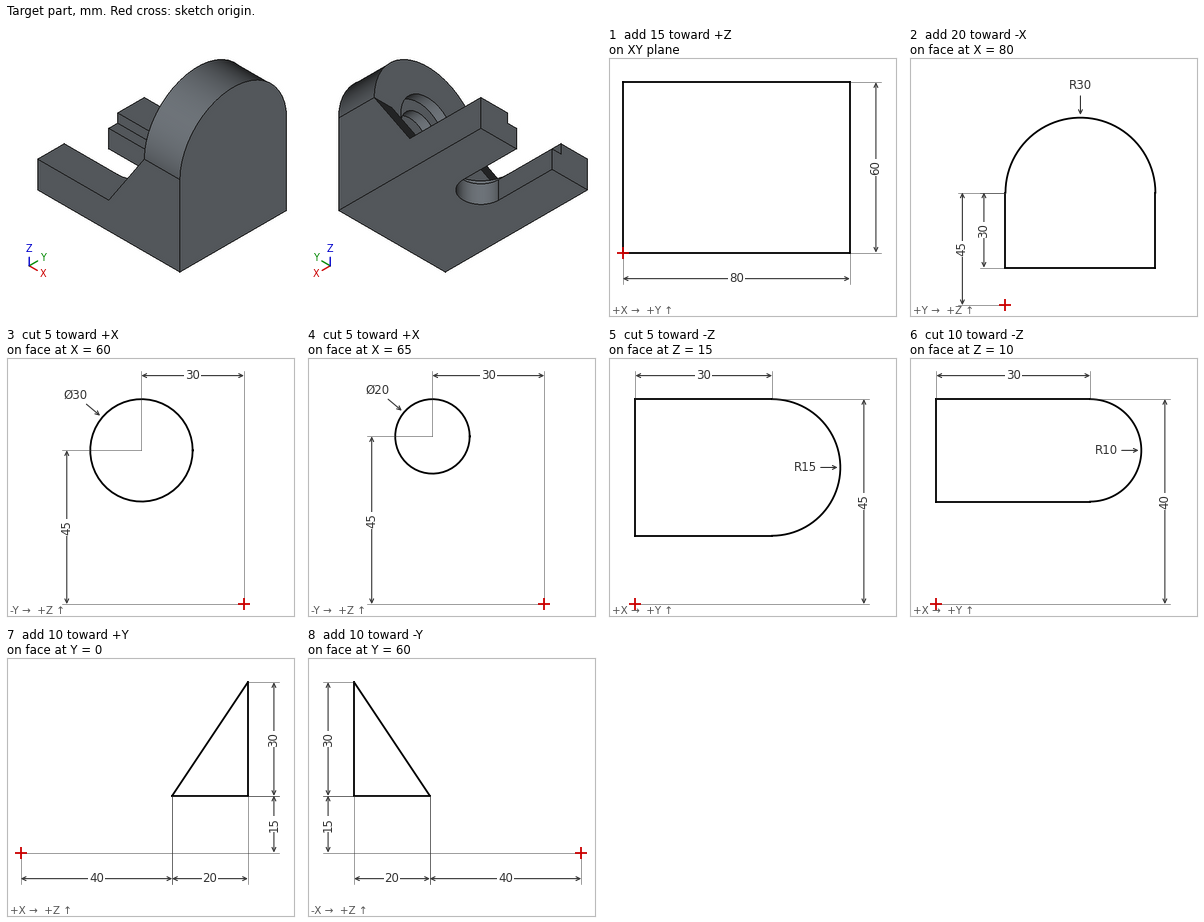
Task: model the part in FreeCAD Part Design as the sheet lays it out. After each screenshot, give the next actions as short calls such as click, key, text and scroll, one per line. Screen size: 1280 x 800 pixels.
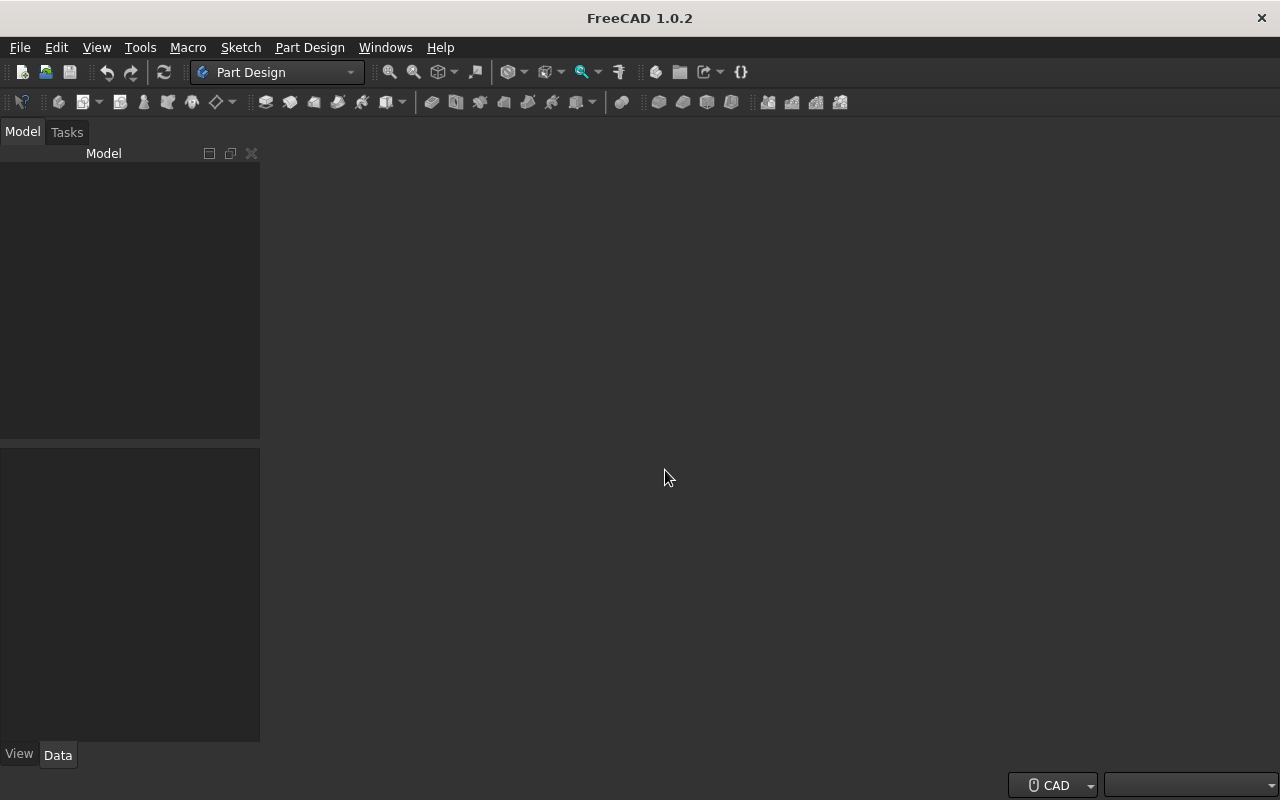
click(22, 72)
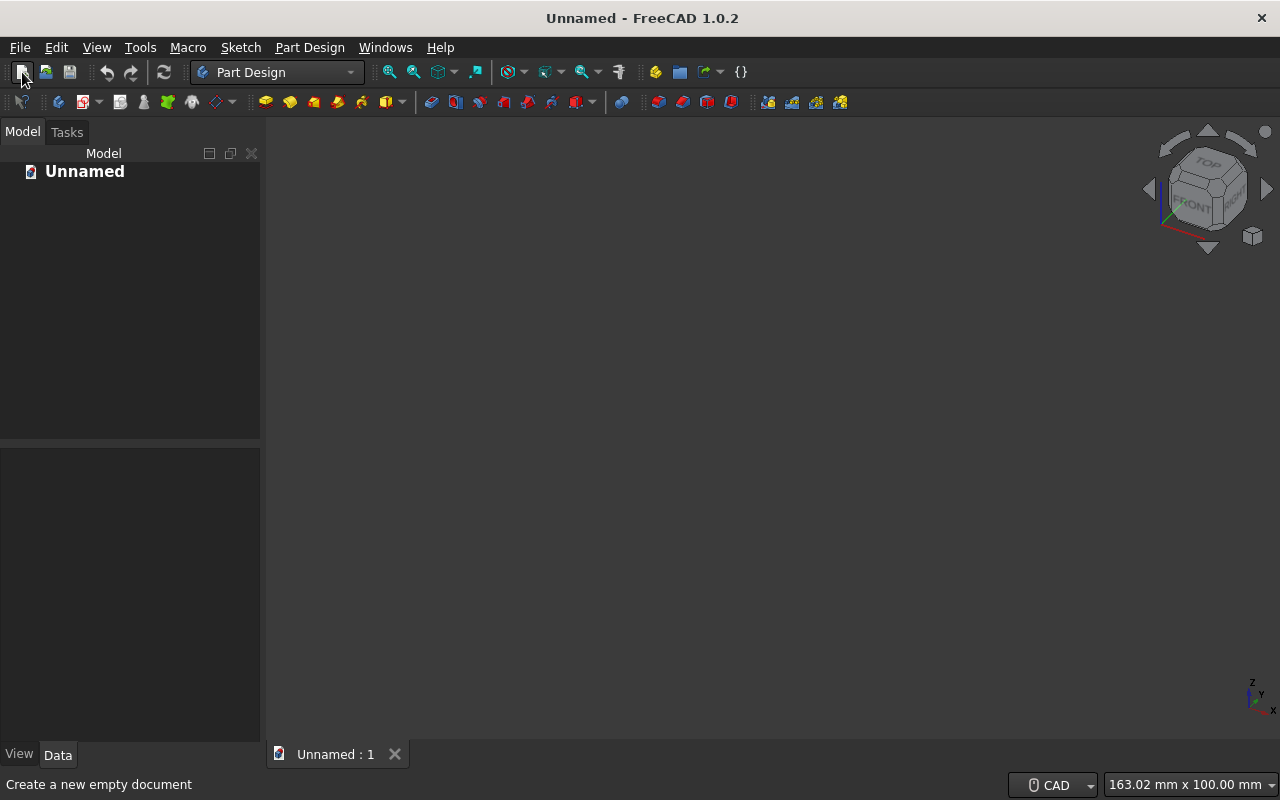
click(84, 102)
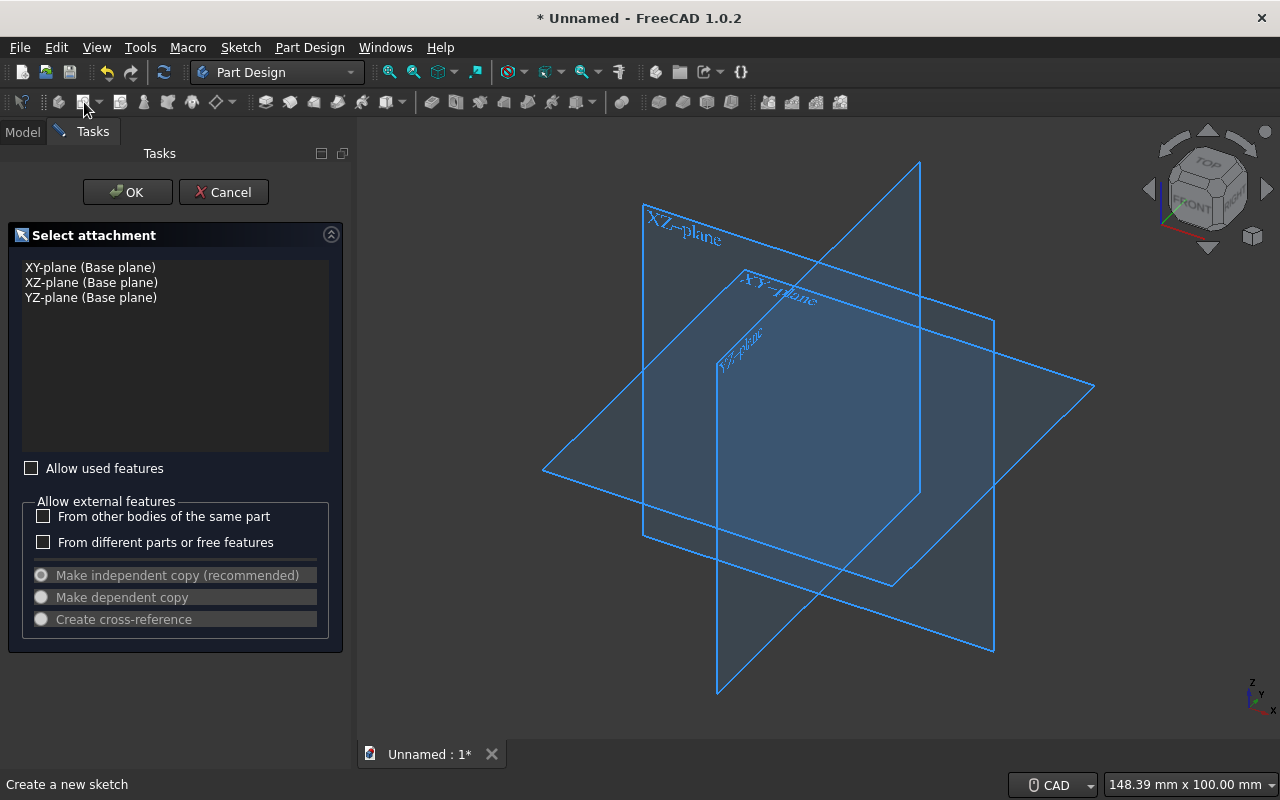
click(82, 268)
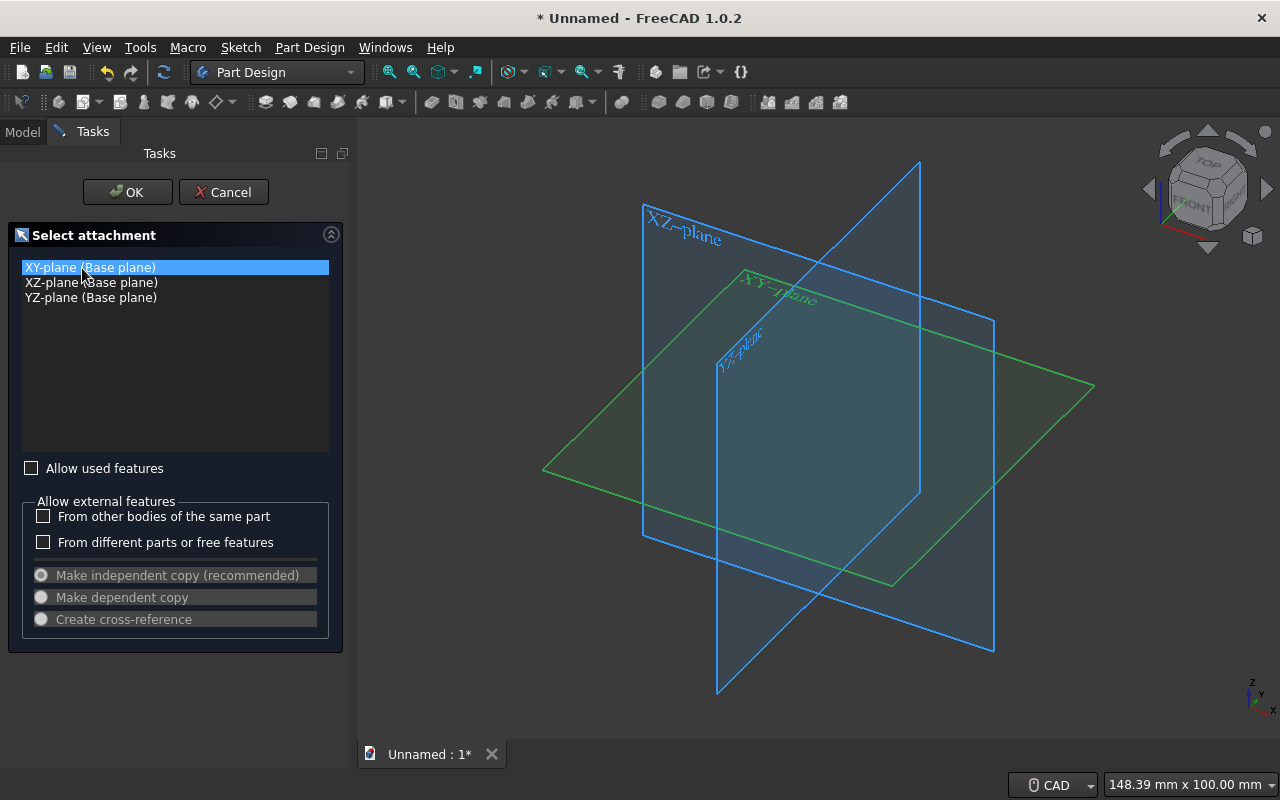
click(128, 192)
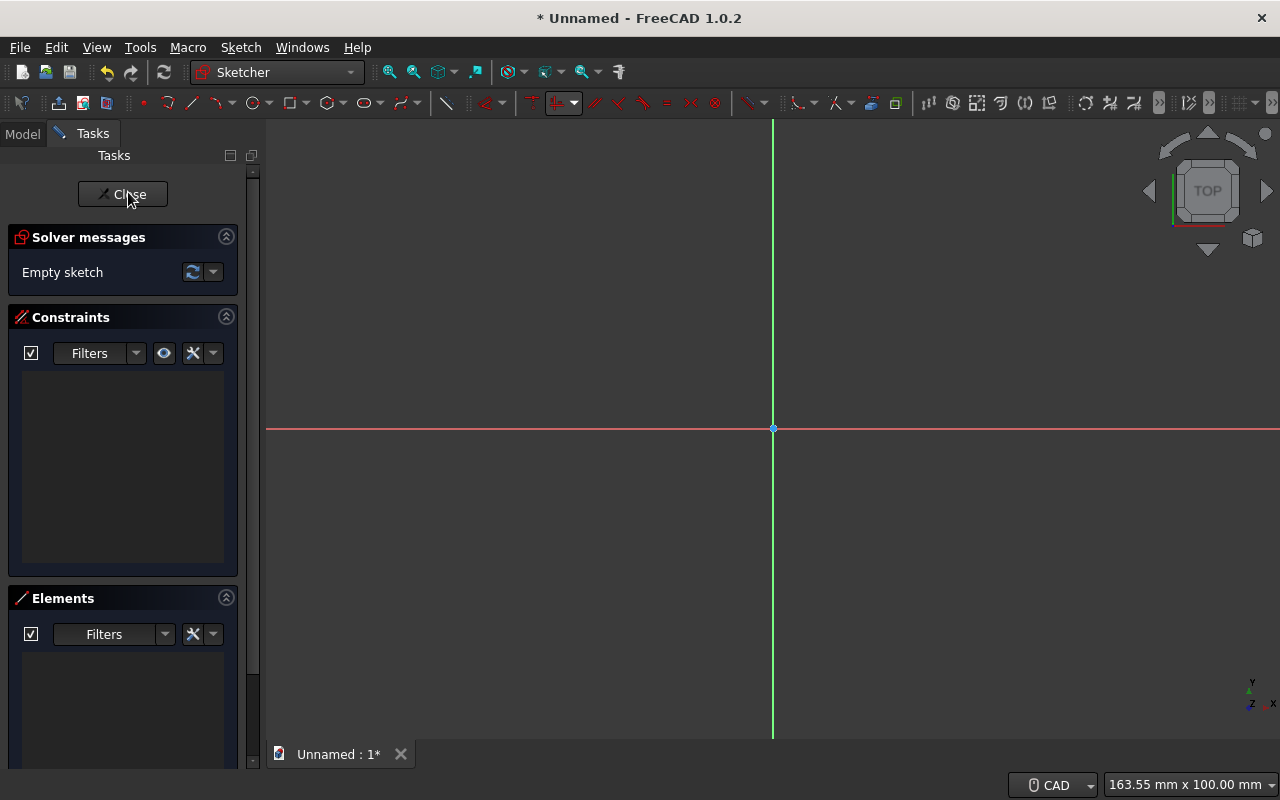
scroll(294, 711, down, 2)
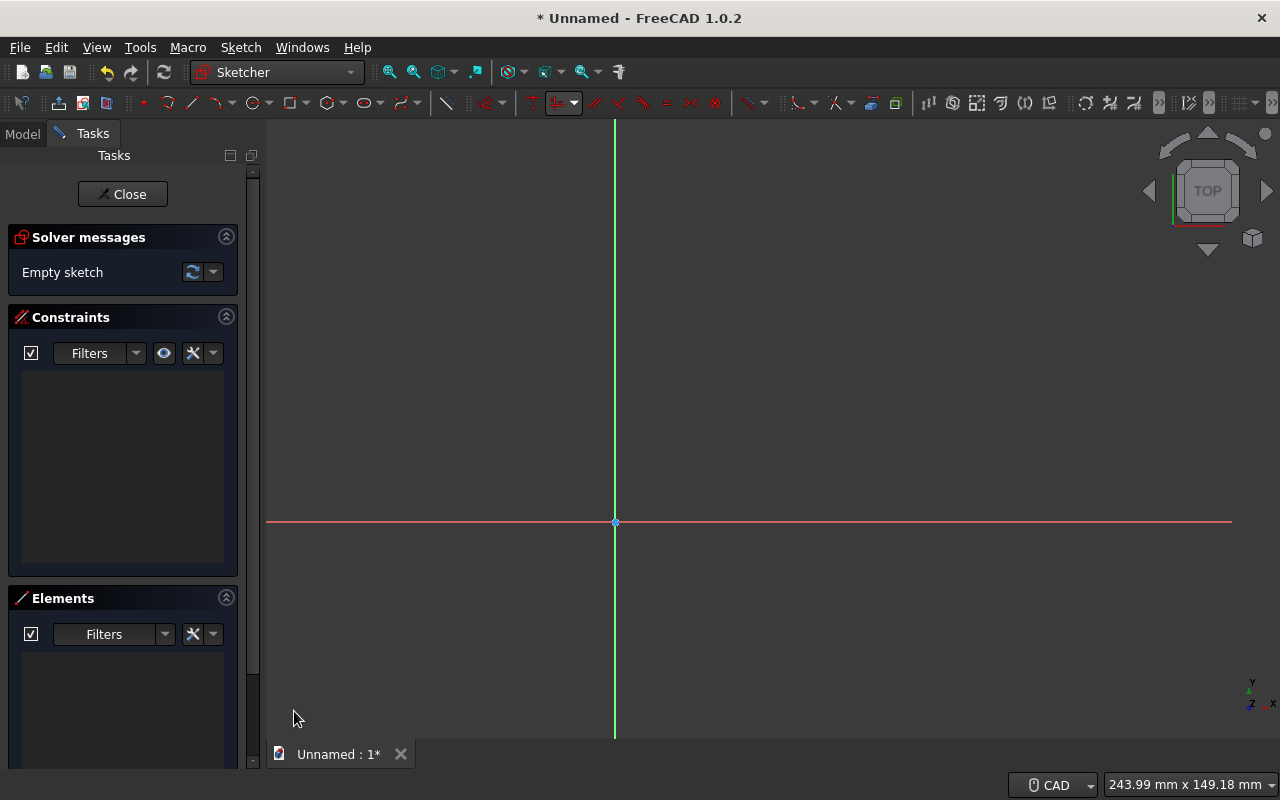
scroll(938, 334, up, 2)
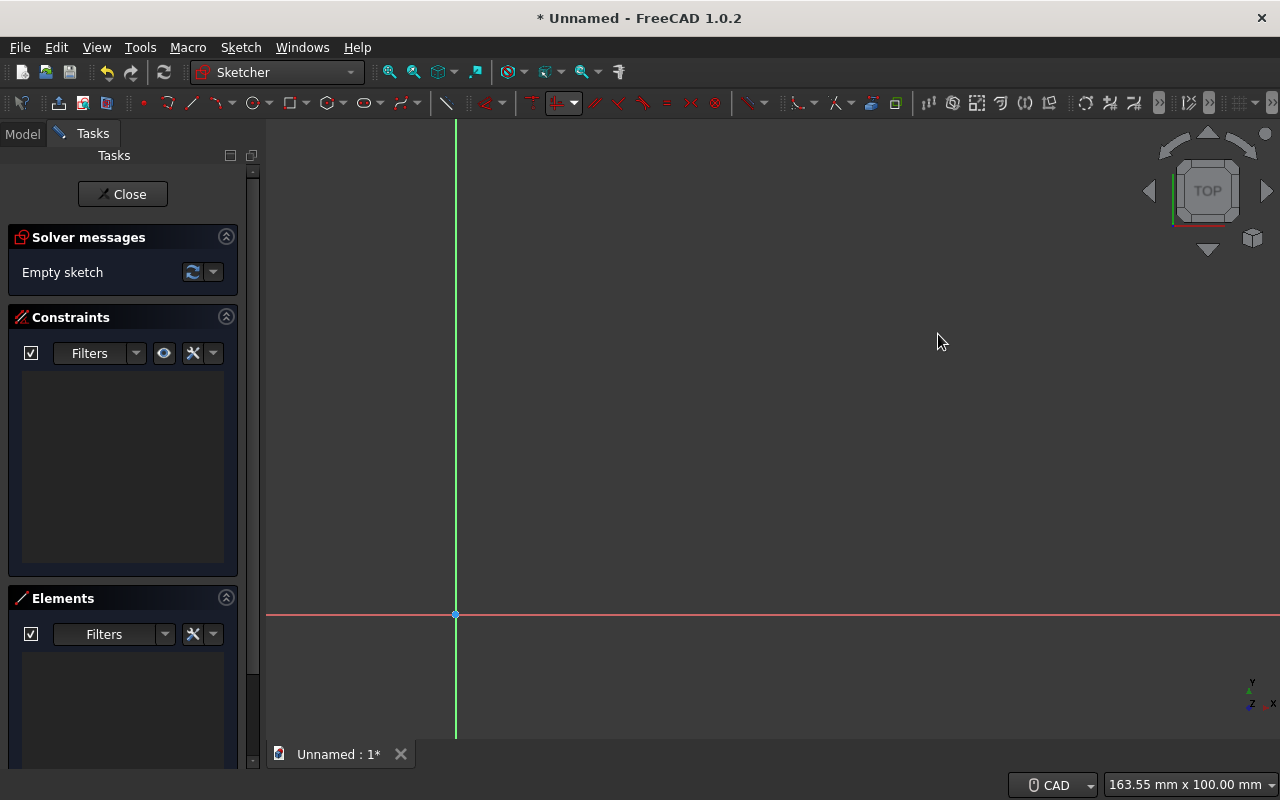
click(290, 104)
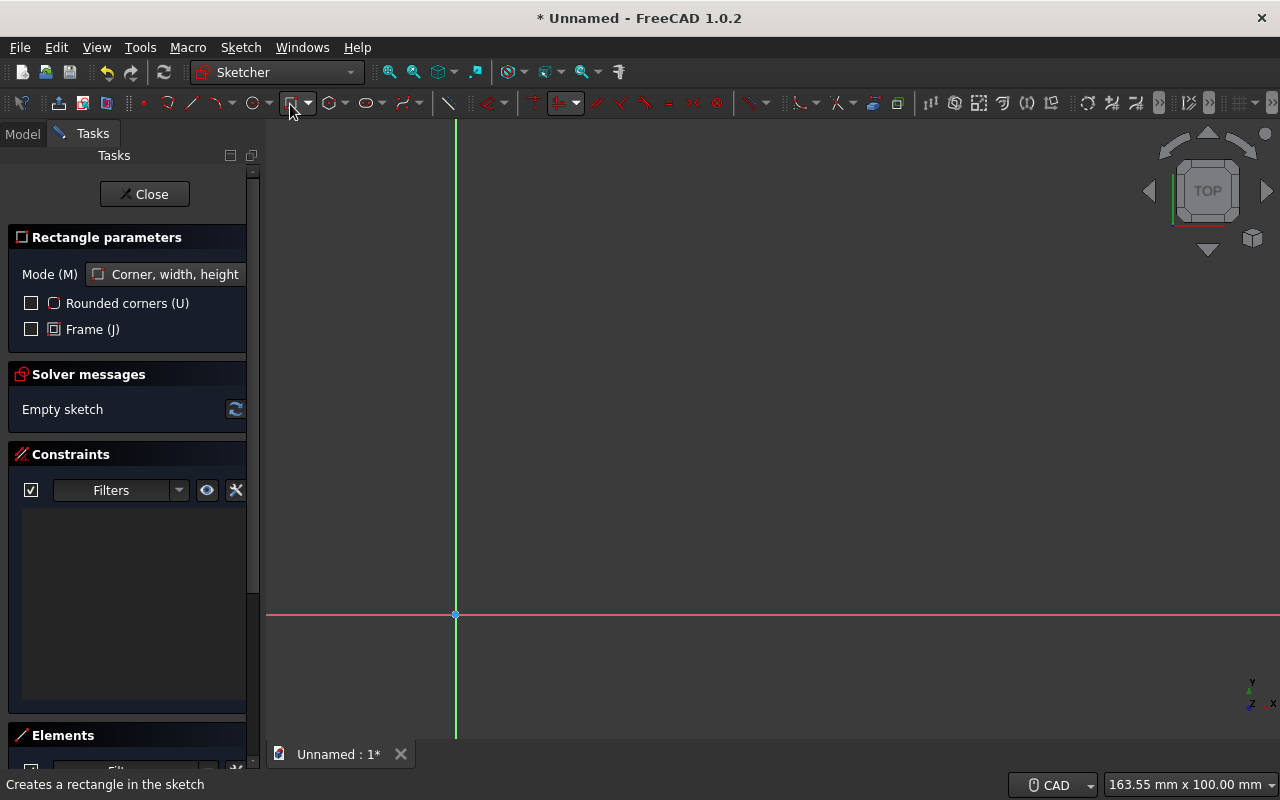
click(456, 615)
click(952, 243)
key(Escape)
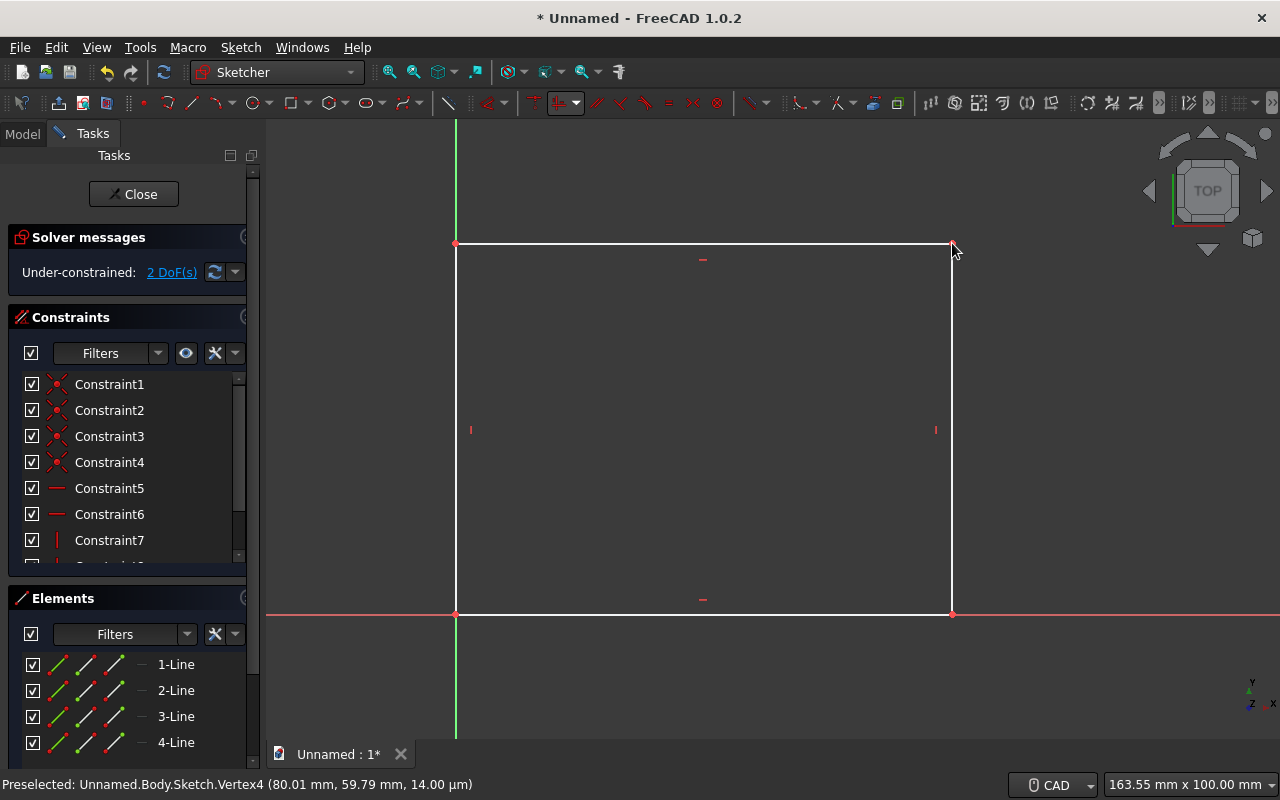
click(488, 104)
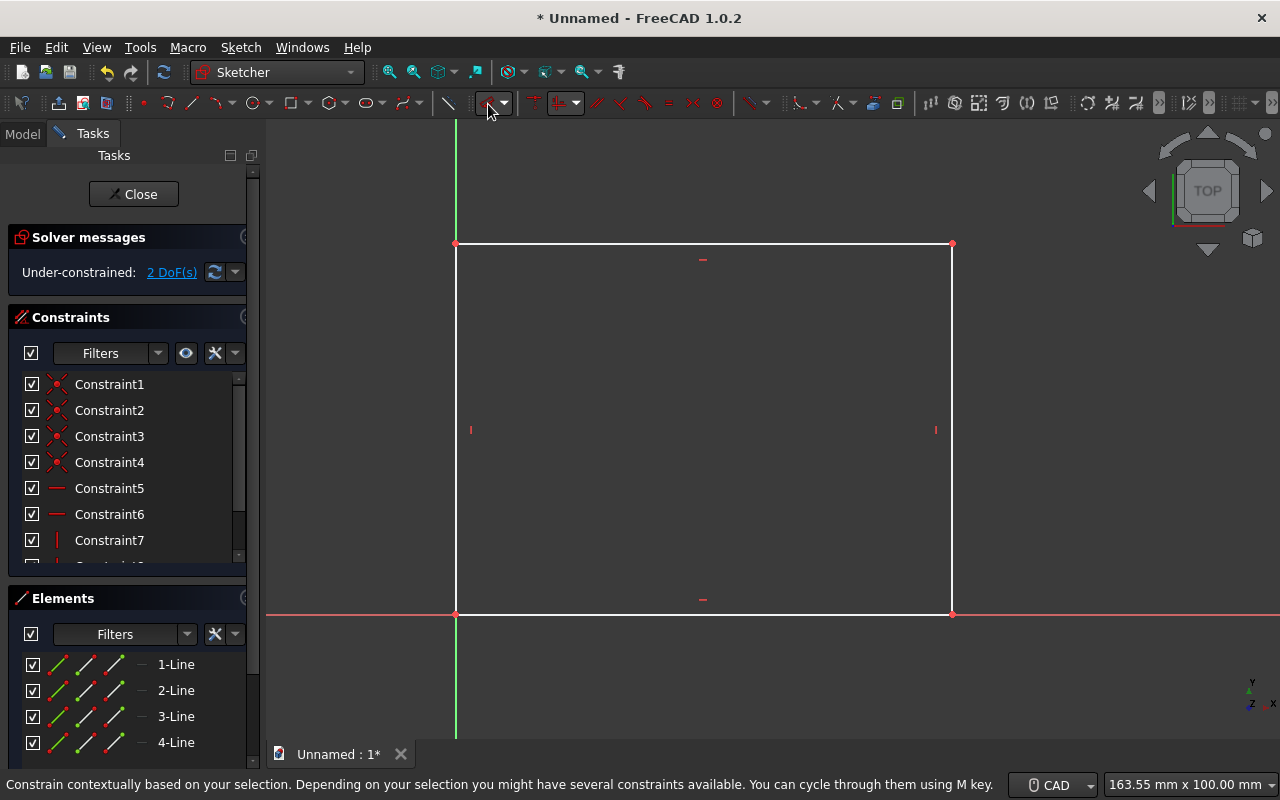
click(605, 615)
click(704, 649)